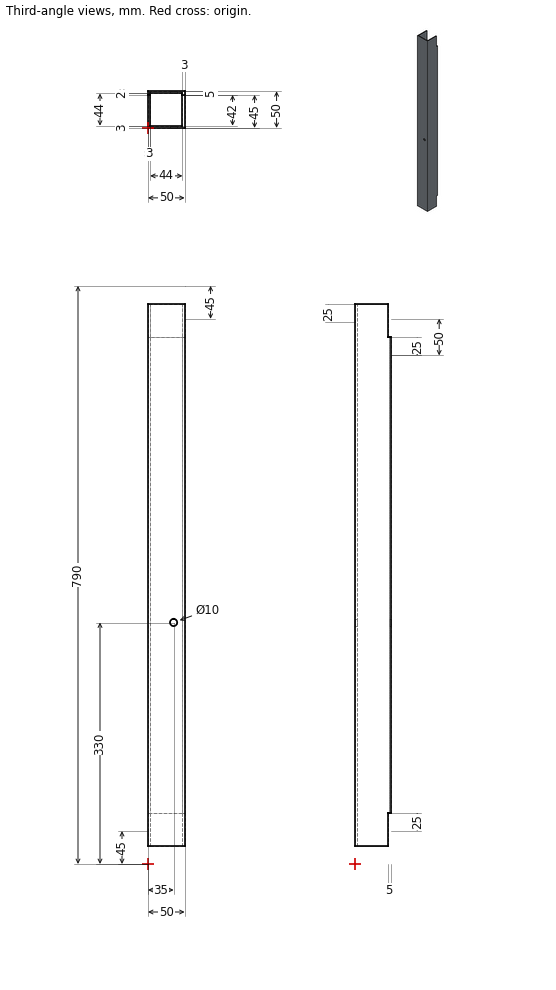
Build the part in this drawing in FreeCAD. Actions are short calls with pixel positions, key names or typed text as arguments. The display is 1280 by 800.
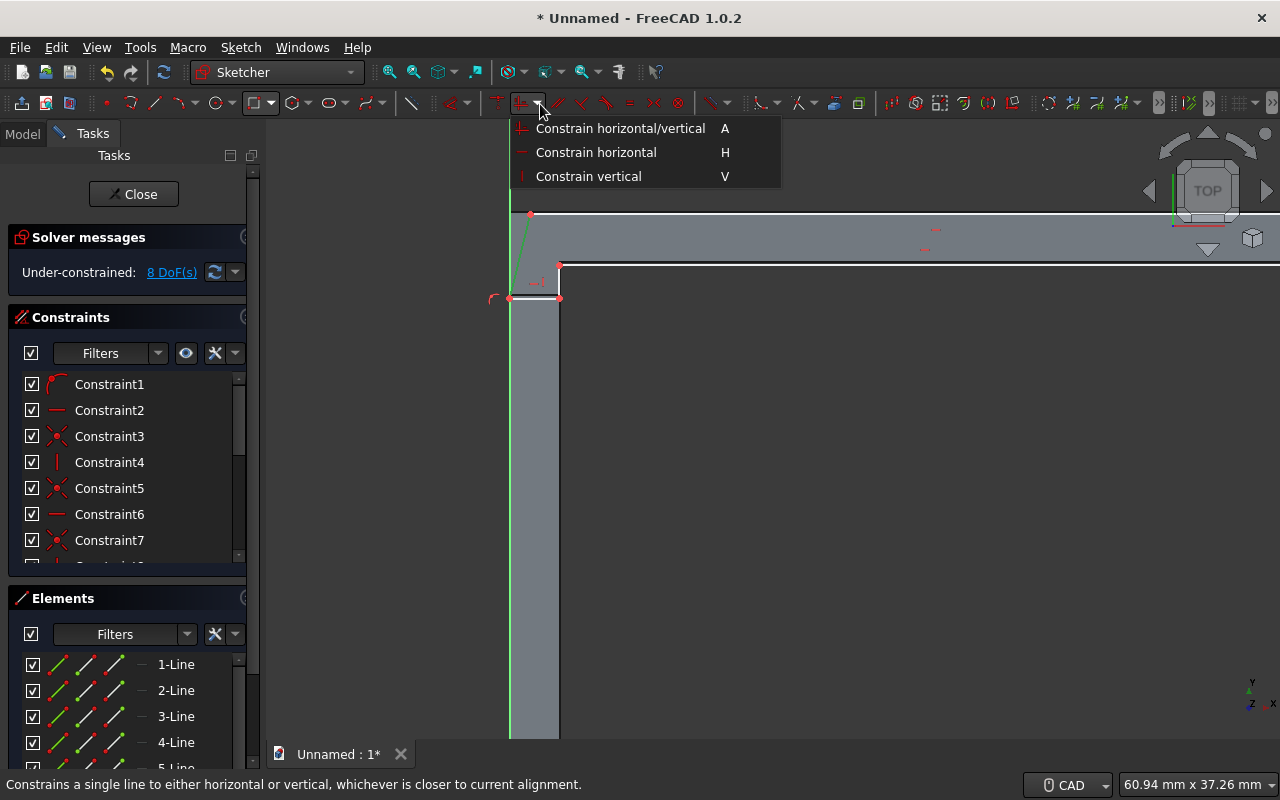
click(646, 176)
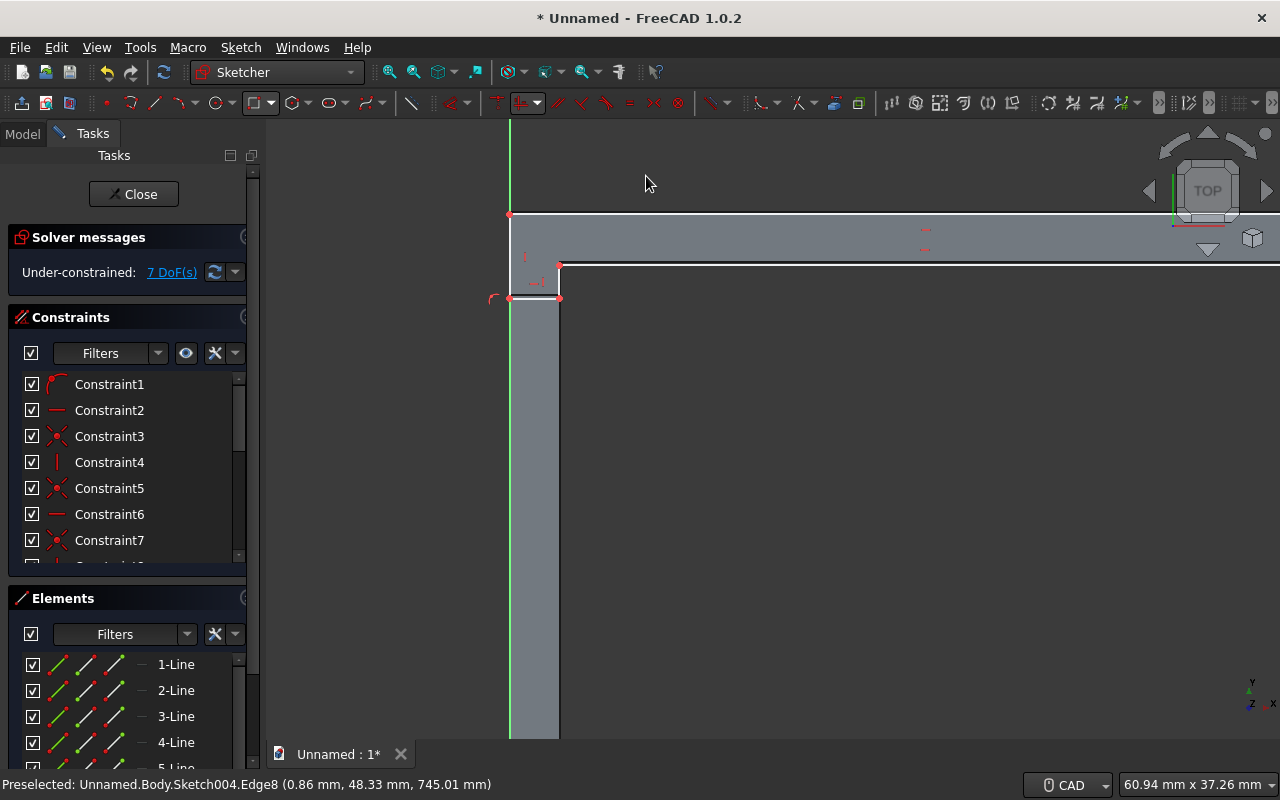
click(450, 104)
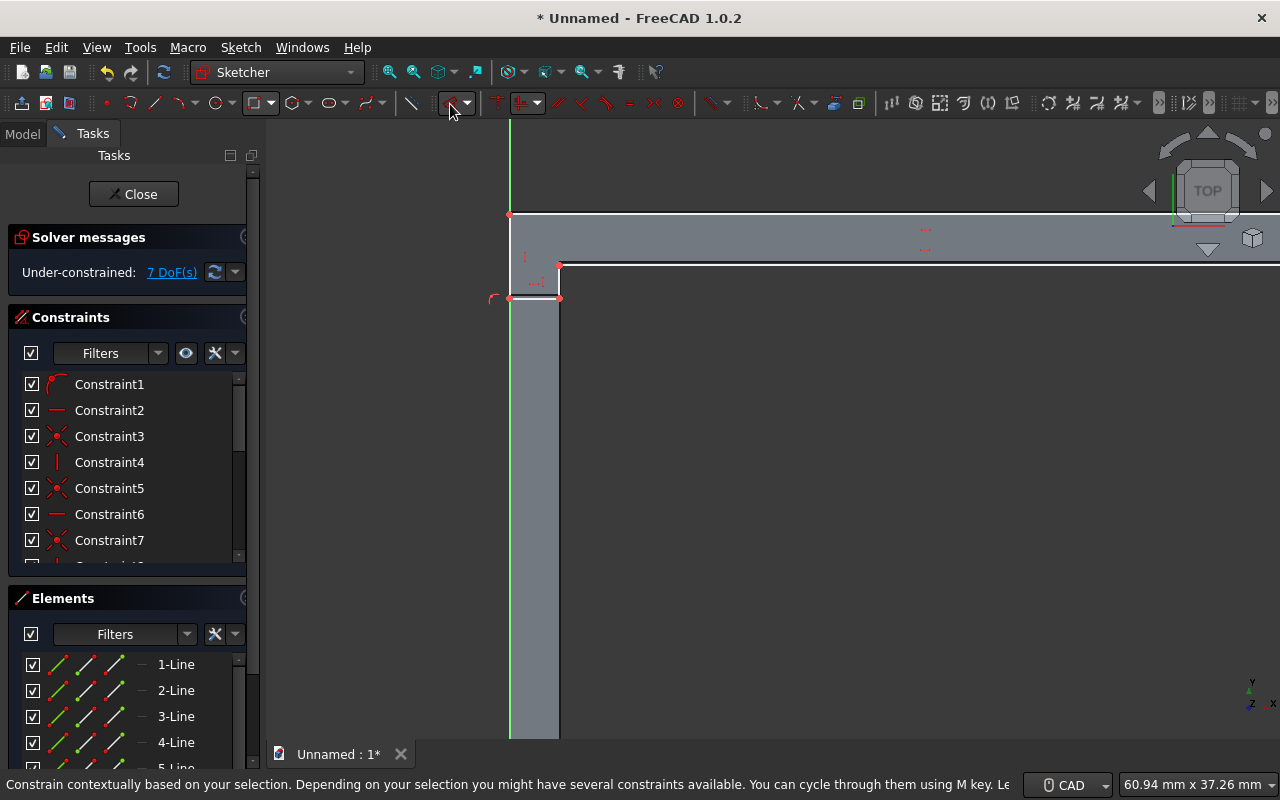
click(525, 299)
click(534, 265)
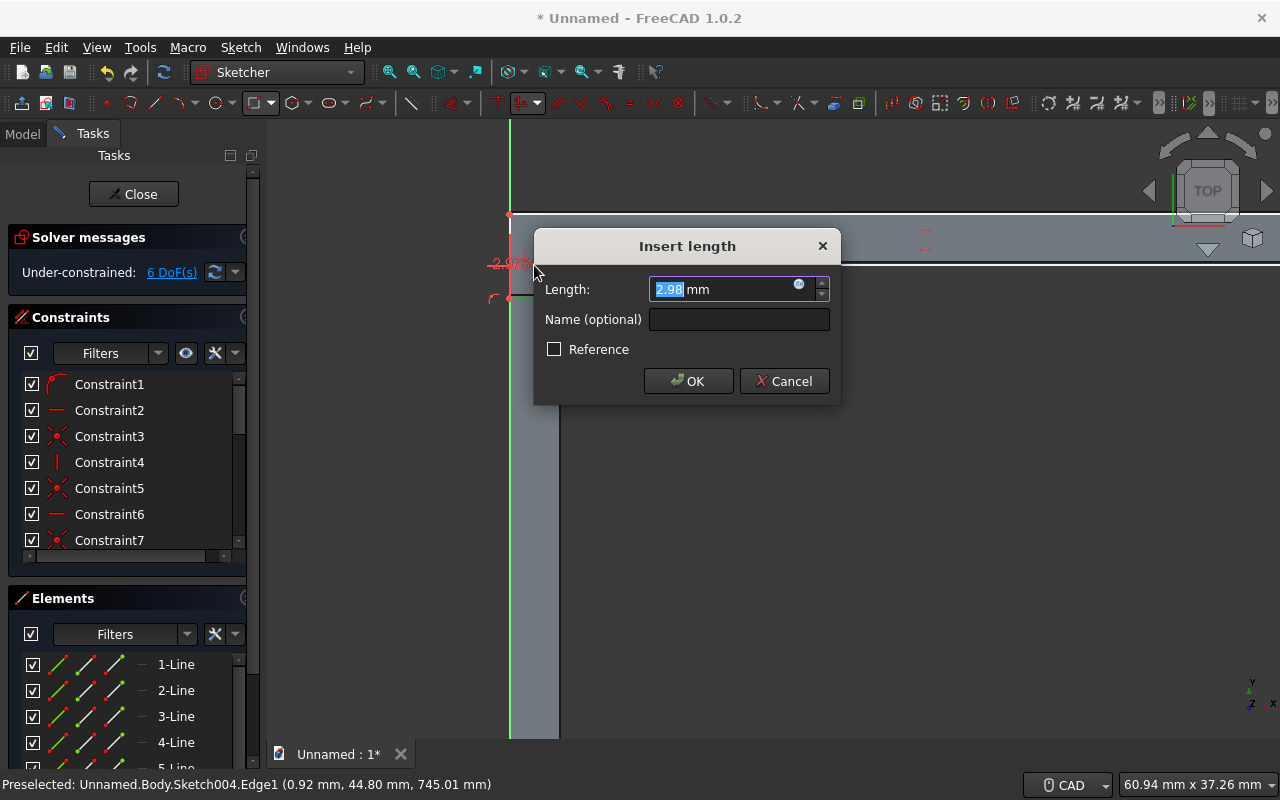
text(3)
key(Return)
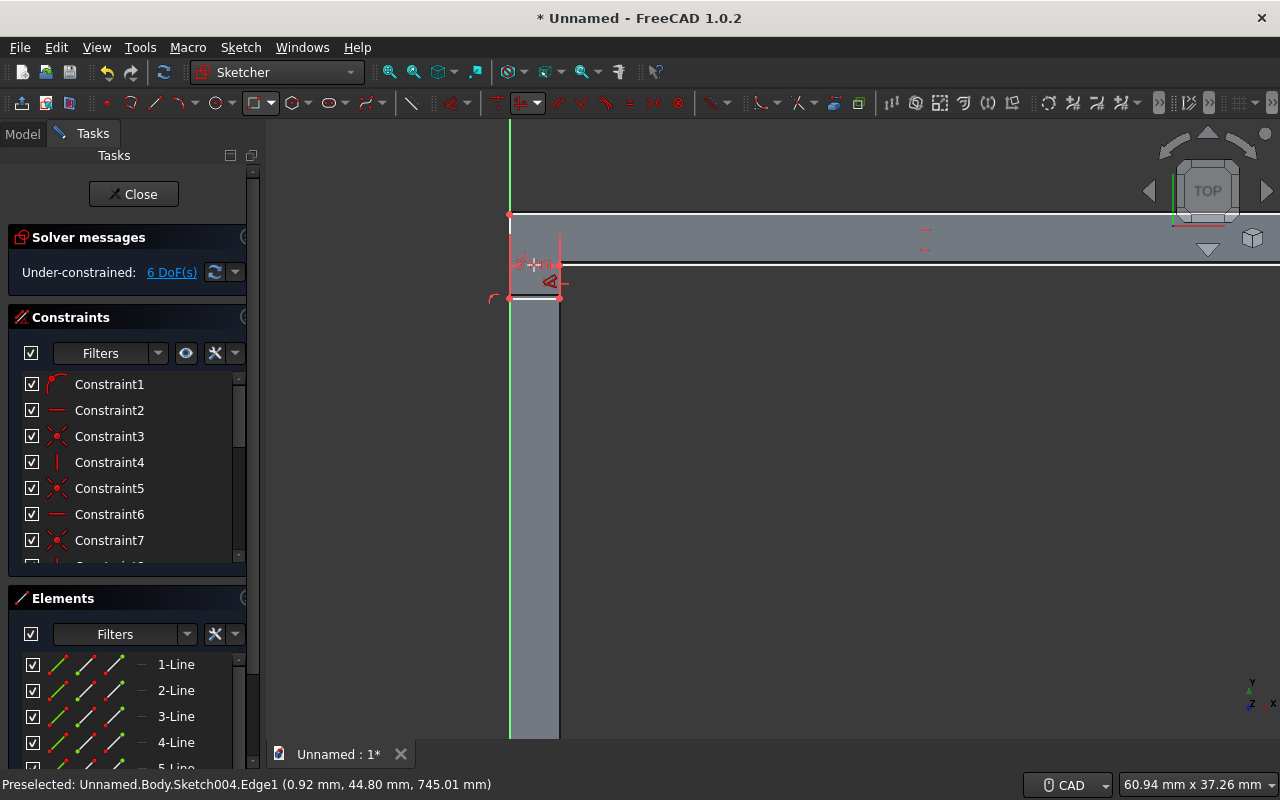
scroll(560, 289, up, 2)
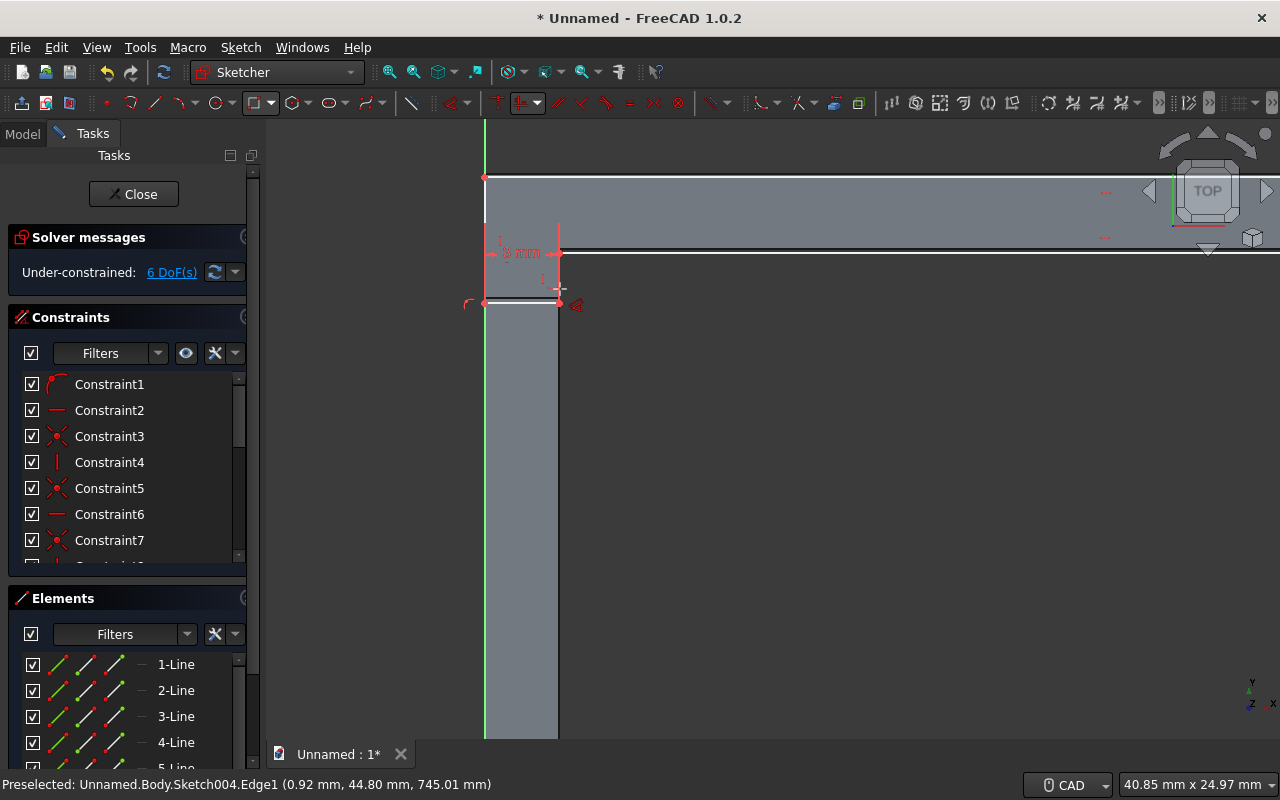
click(559, 288)
click(525, 278)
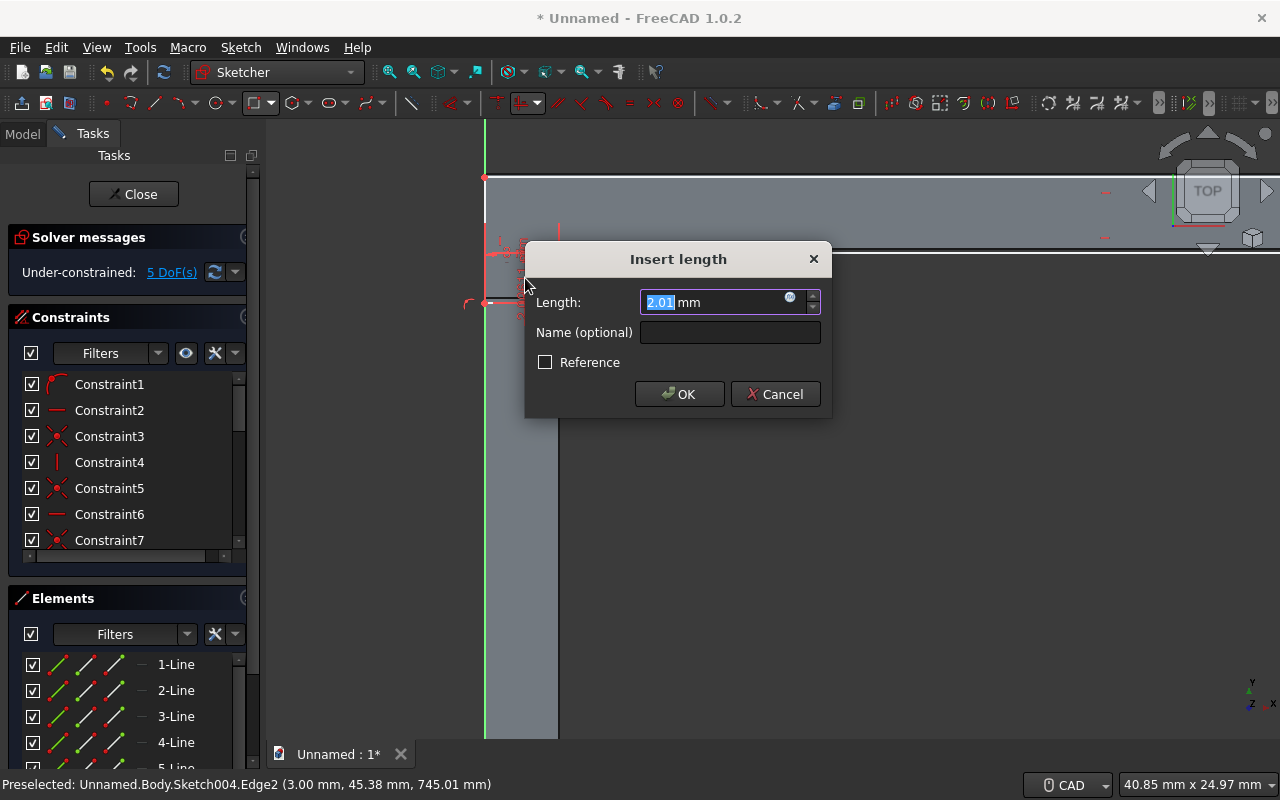
text(2)
key(Return)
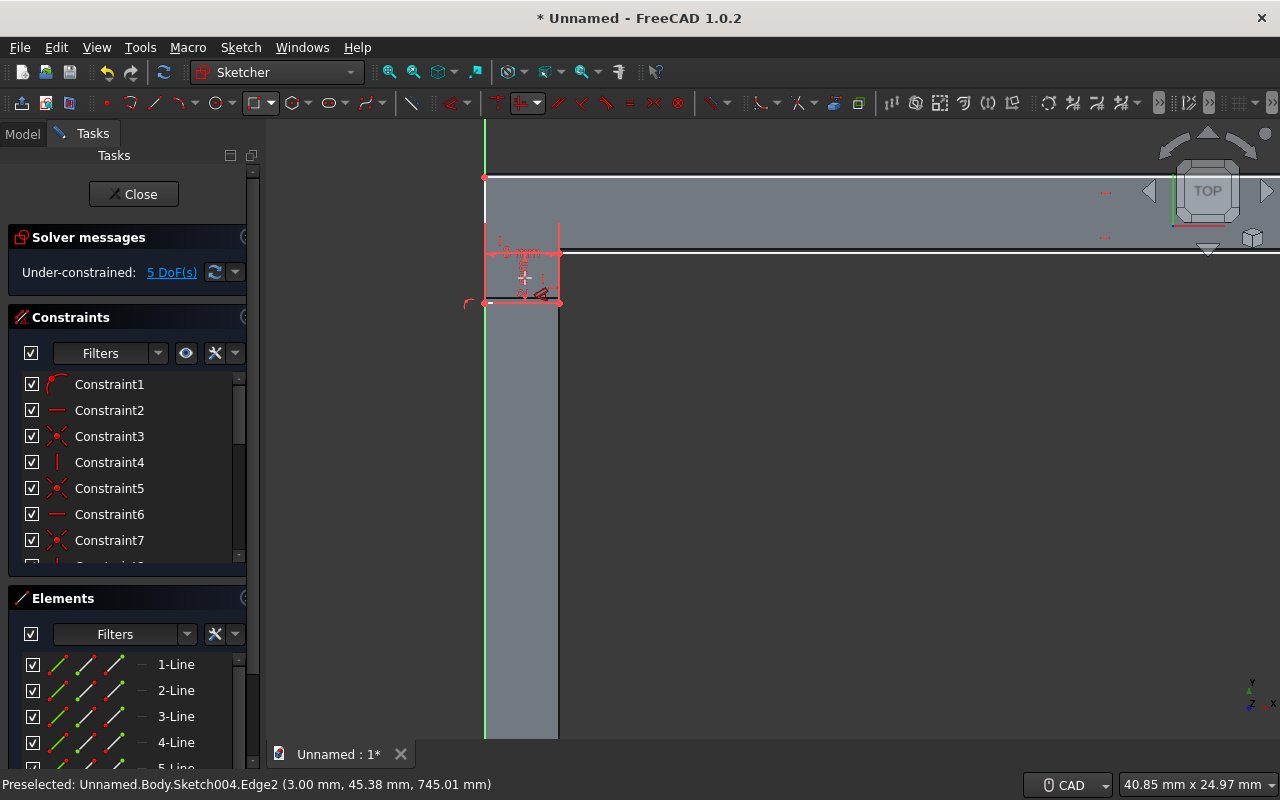
scroll(532, 271, down, 6)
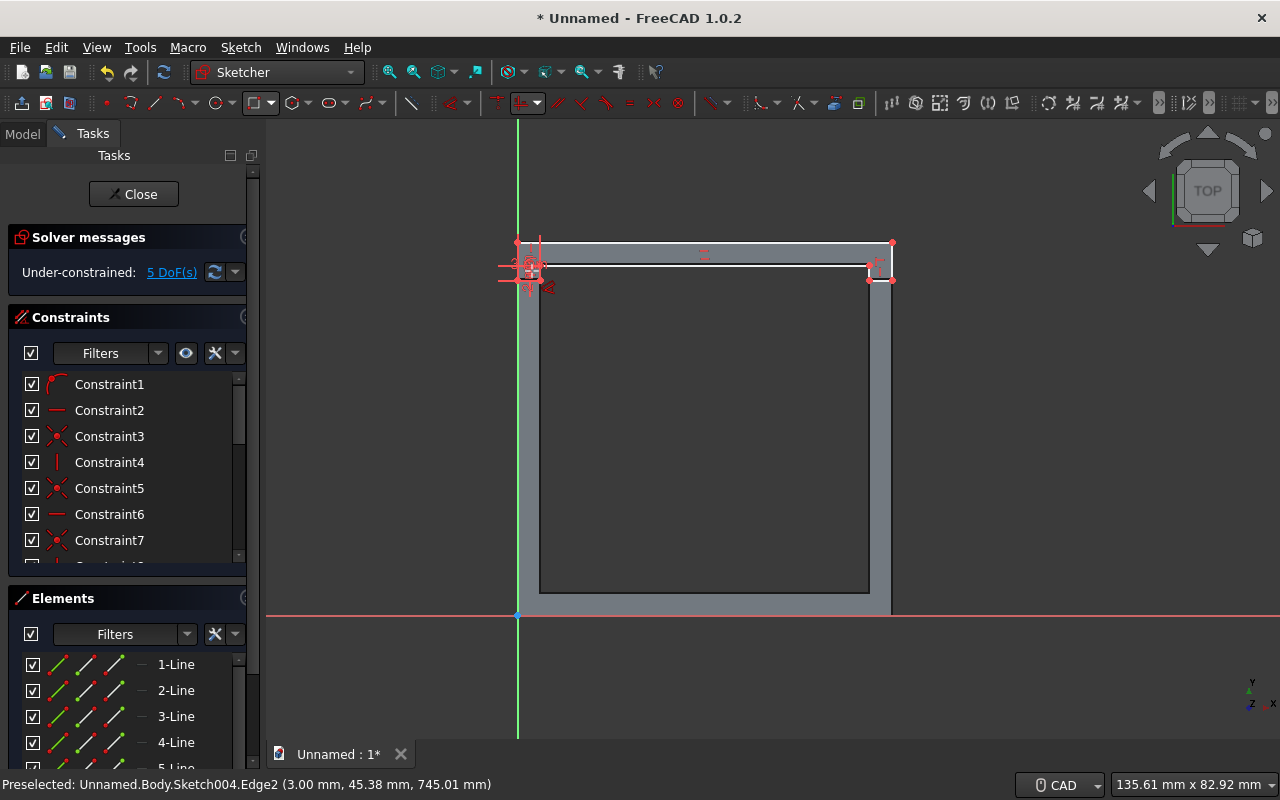
scroll(869, 270, up, 6)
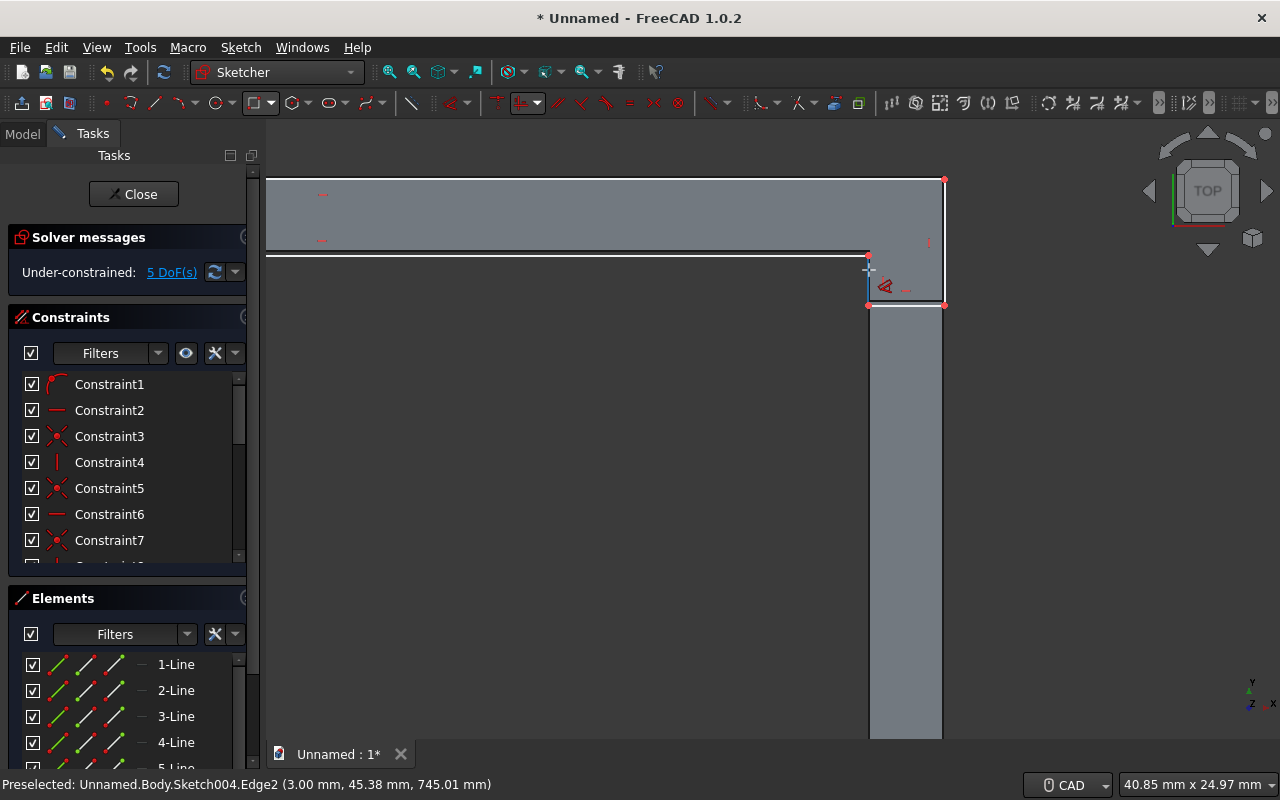
click(868, 271)
click(902, 281)